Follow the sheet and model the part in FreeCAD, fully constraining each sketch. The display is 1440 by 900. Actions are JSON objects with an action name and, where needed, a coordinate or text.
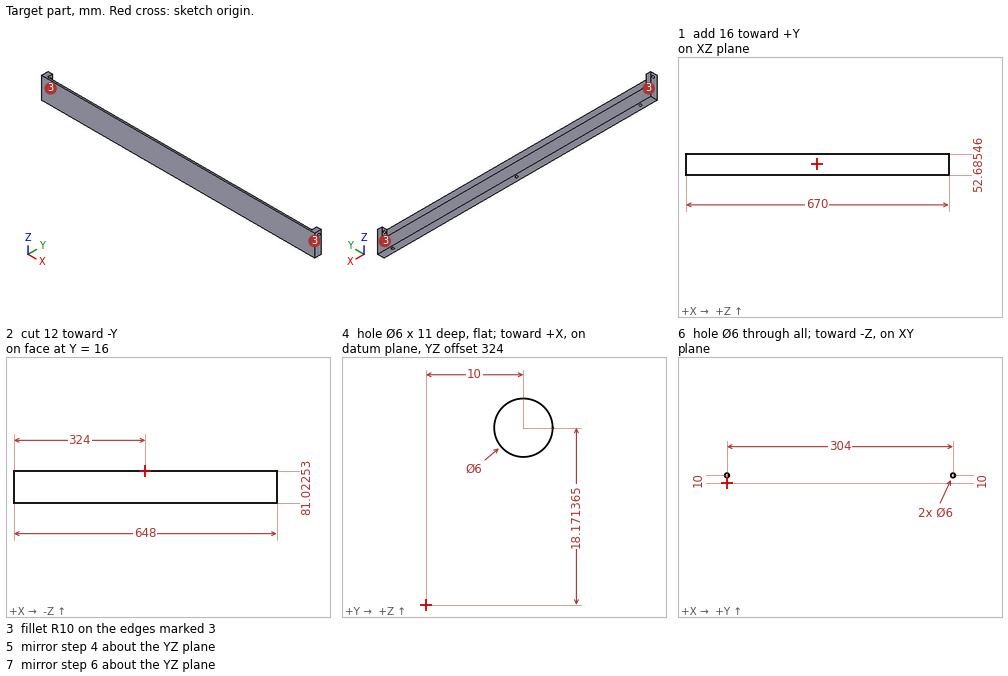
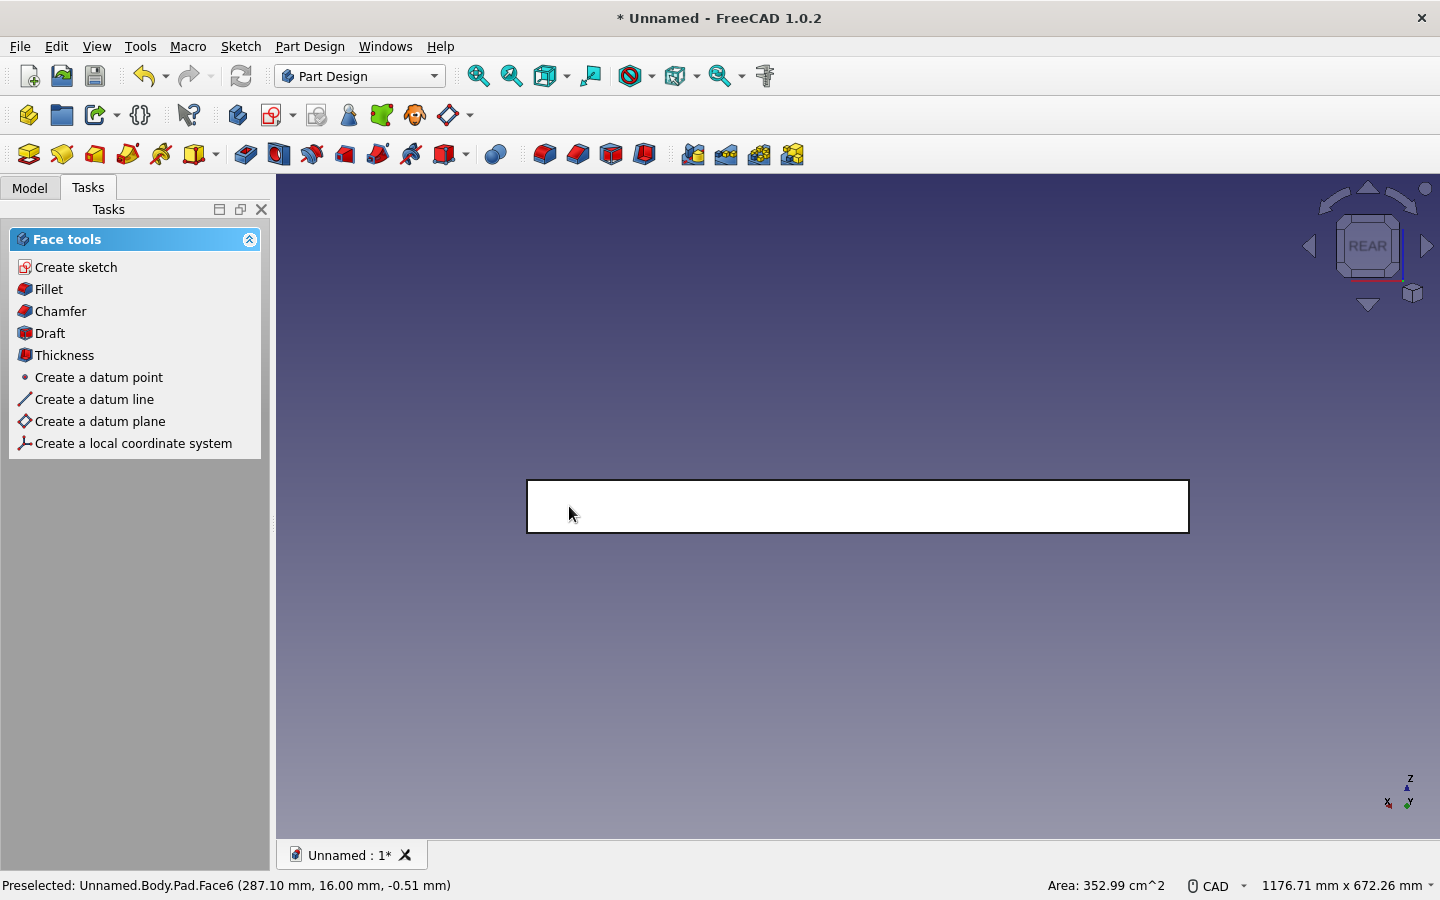
{"action": "left_click", "coordinate": [270, 116]}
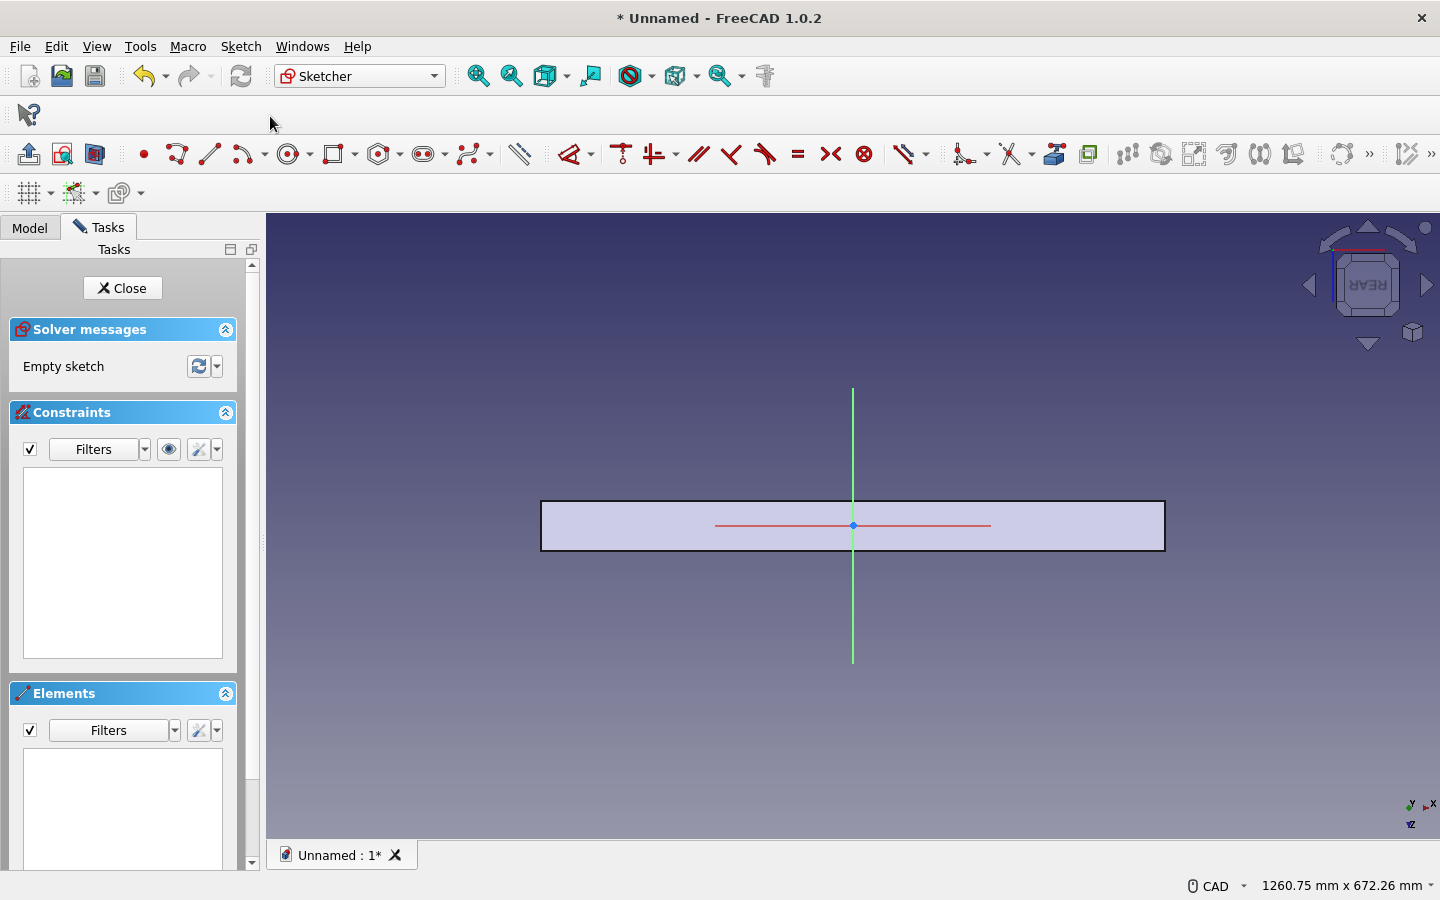
{"action": "left_click", "coordinate": [332, 154]}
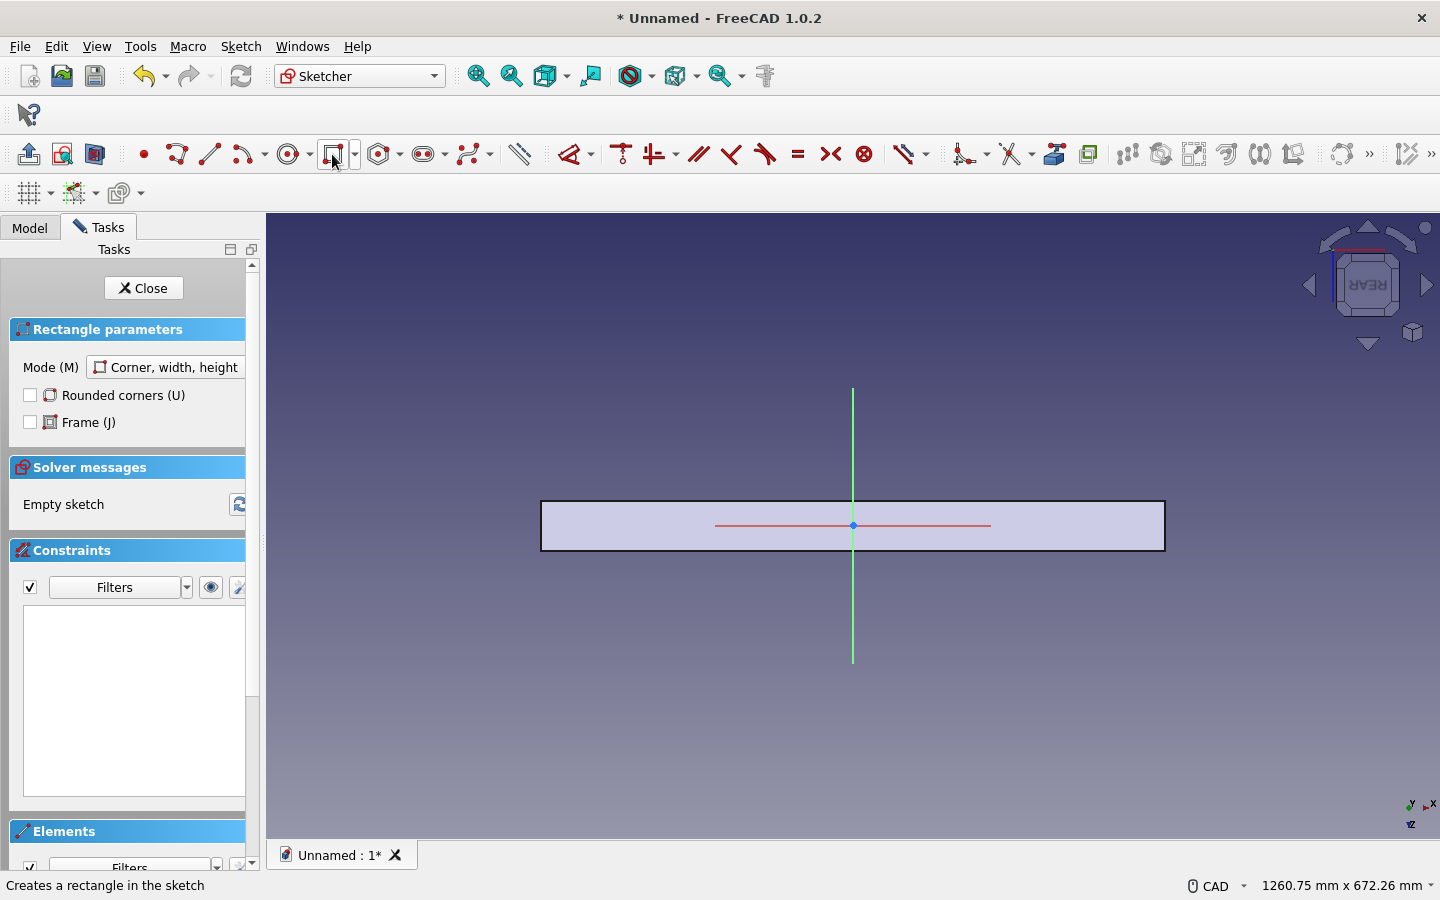
{"action": "left_click", "coordinate": [551, 526]}
{"action": "mouse_move", "coordinate": [1155, 601]}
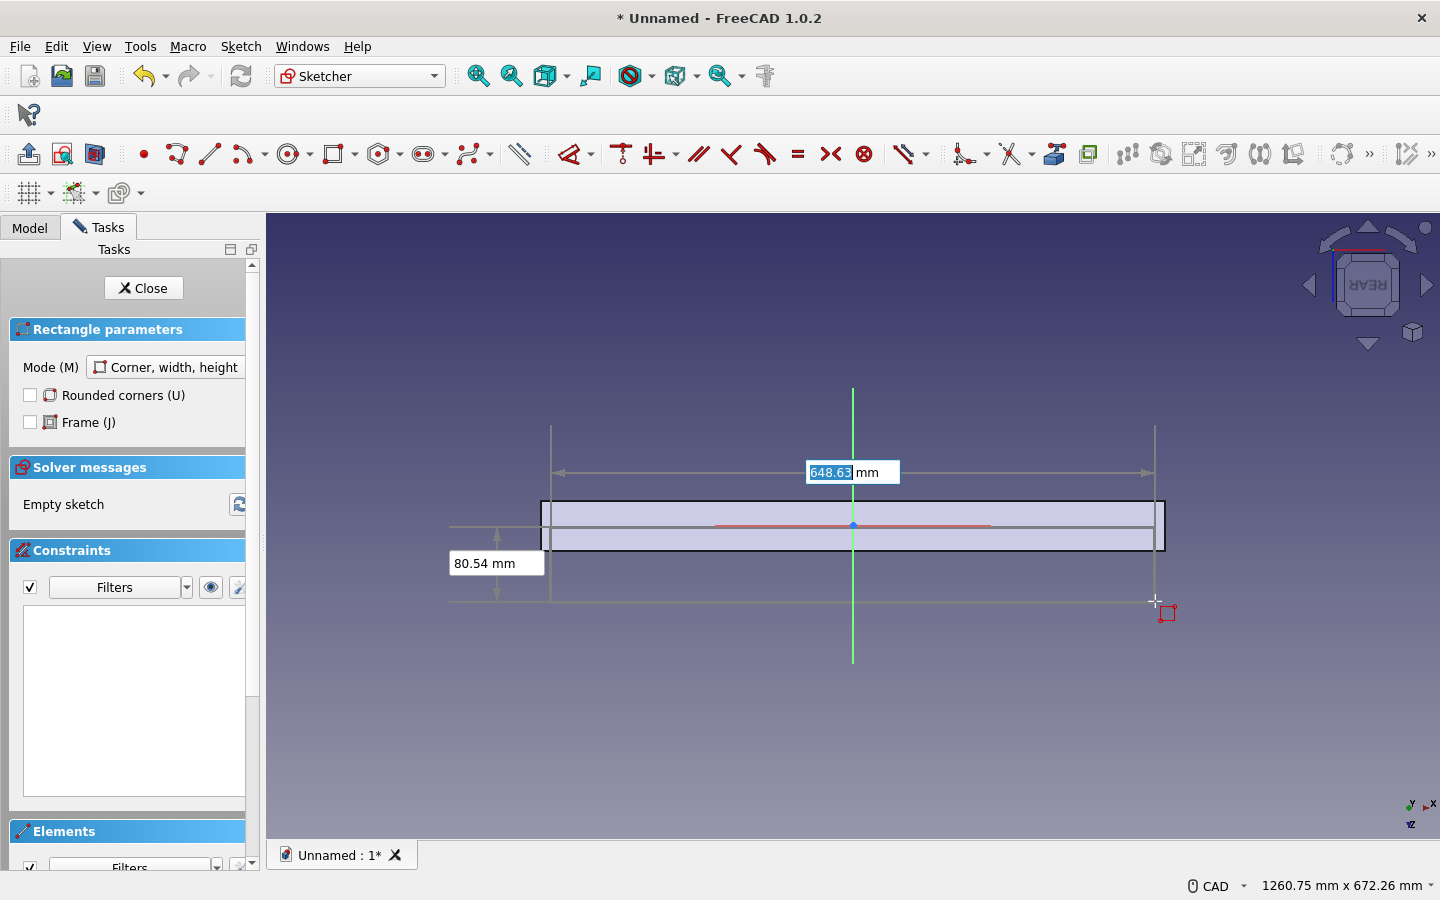
{"action": "type", "text": "648"}
{"action": "key", "text": "Tab"}
{"action": "type", "text": "81.02253"}
{"action": "key", "text": "Return"}
{"action": "key", "text": "Escape"}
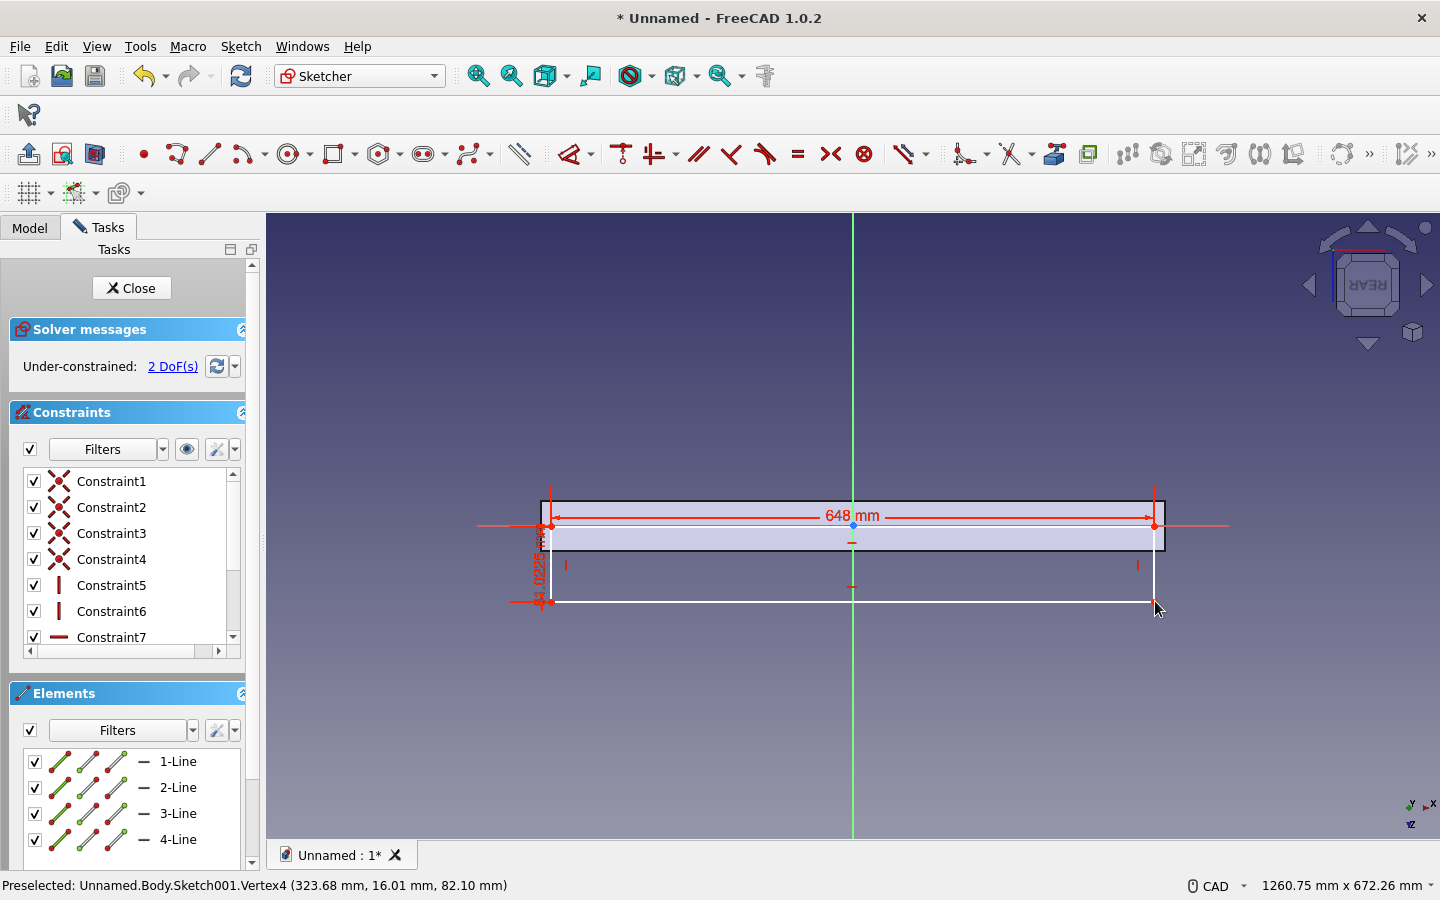
{"action": "left_click", "coordinate": [551, 527]}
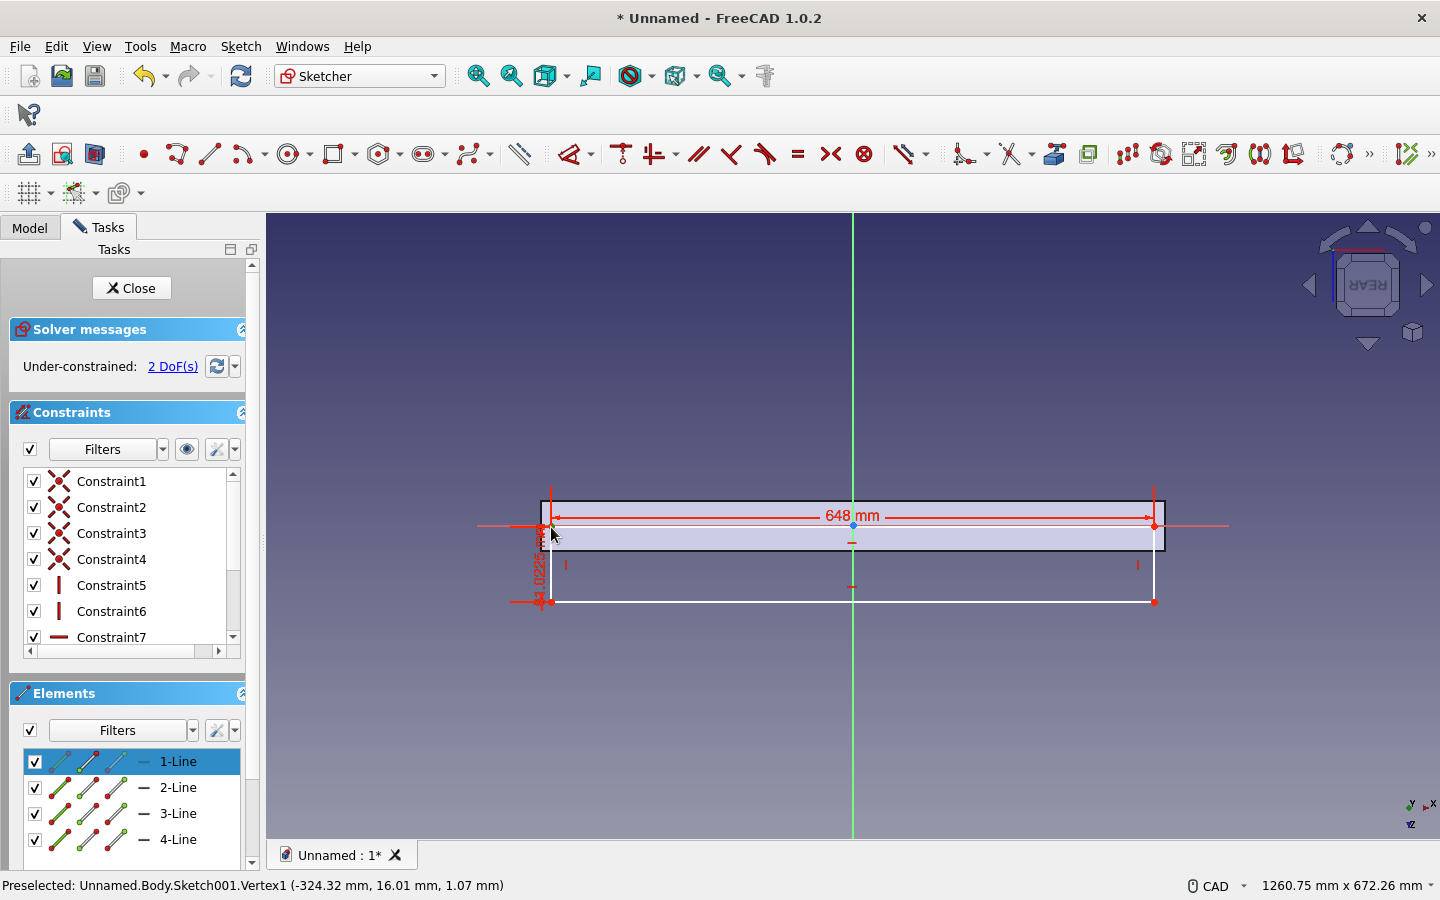
{"action": "left_click", "coordinate": [504, 526]}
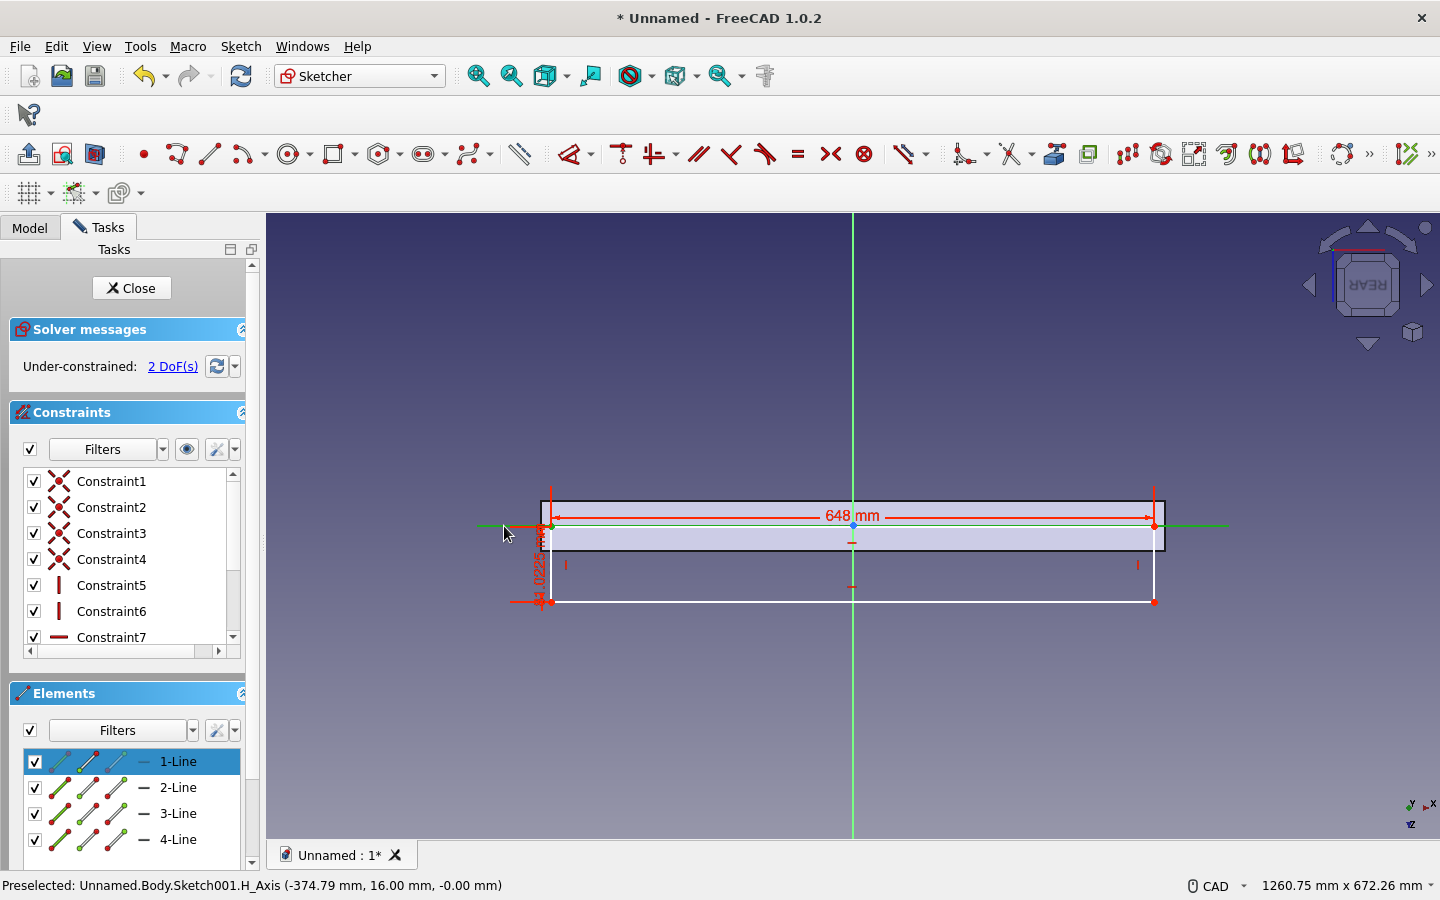
{"action": "left_click", "coordinate": [621, 154]}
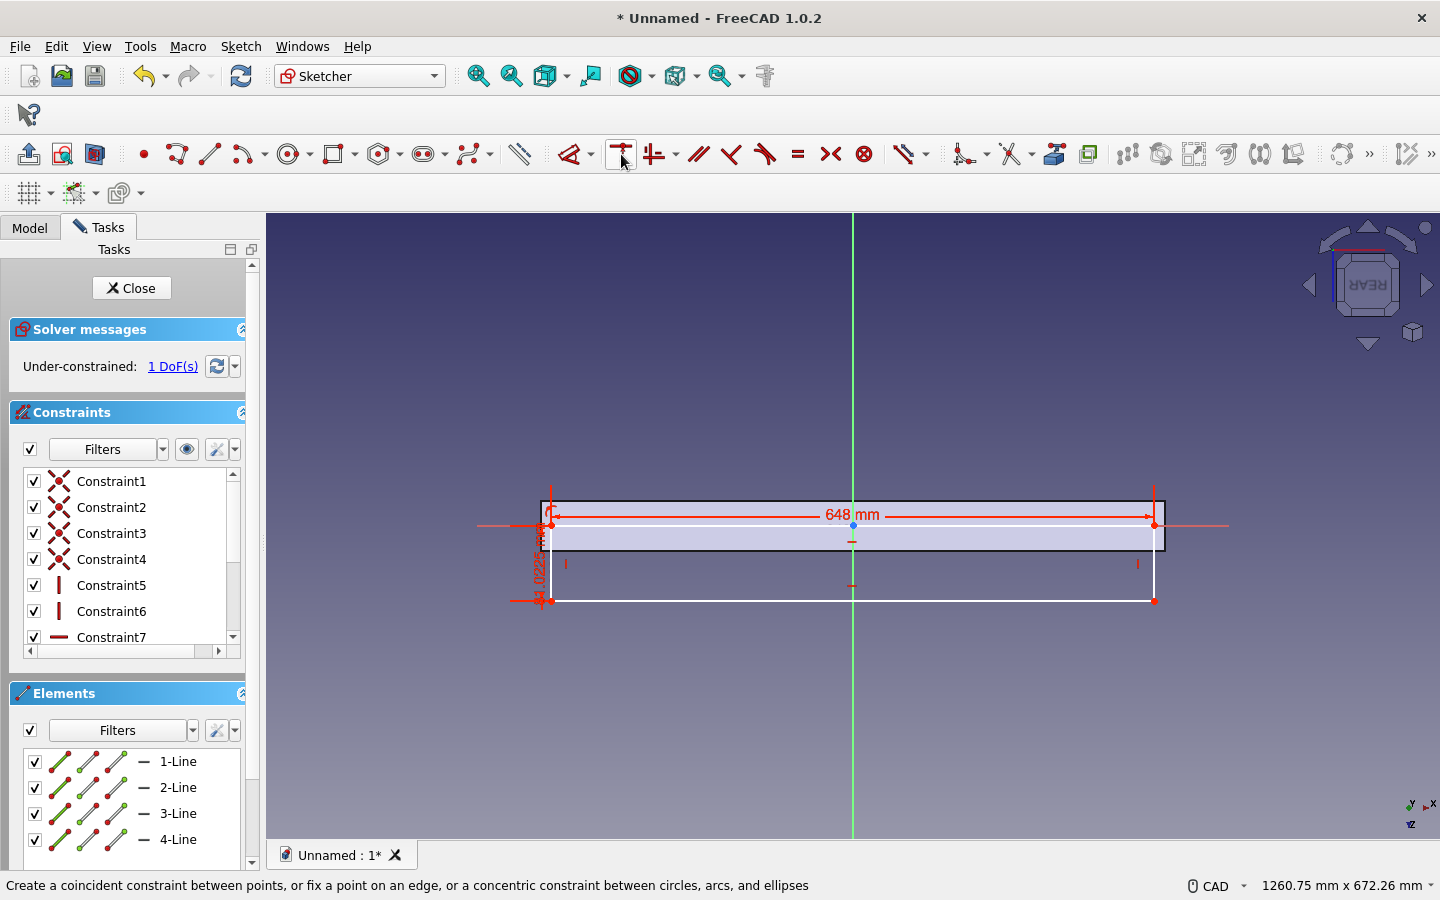
{"action": "left_click", "coordinate": [551, 526]}